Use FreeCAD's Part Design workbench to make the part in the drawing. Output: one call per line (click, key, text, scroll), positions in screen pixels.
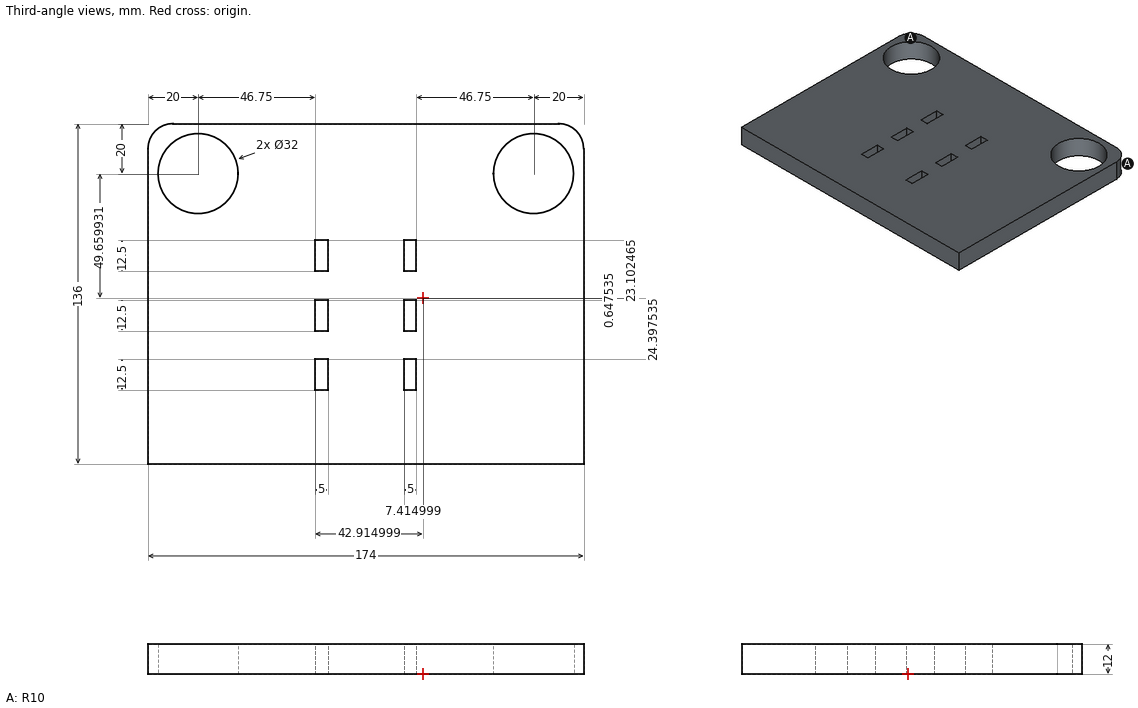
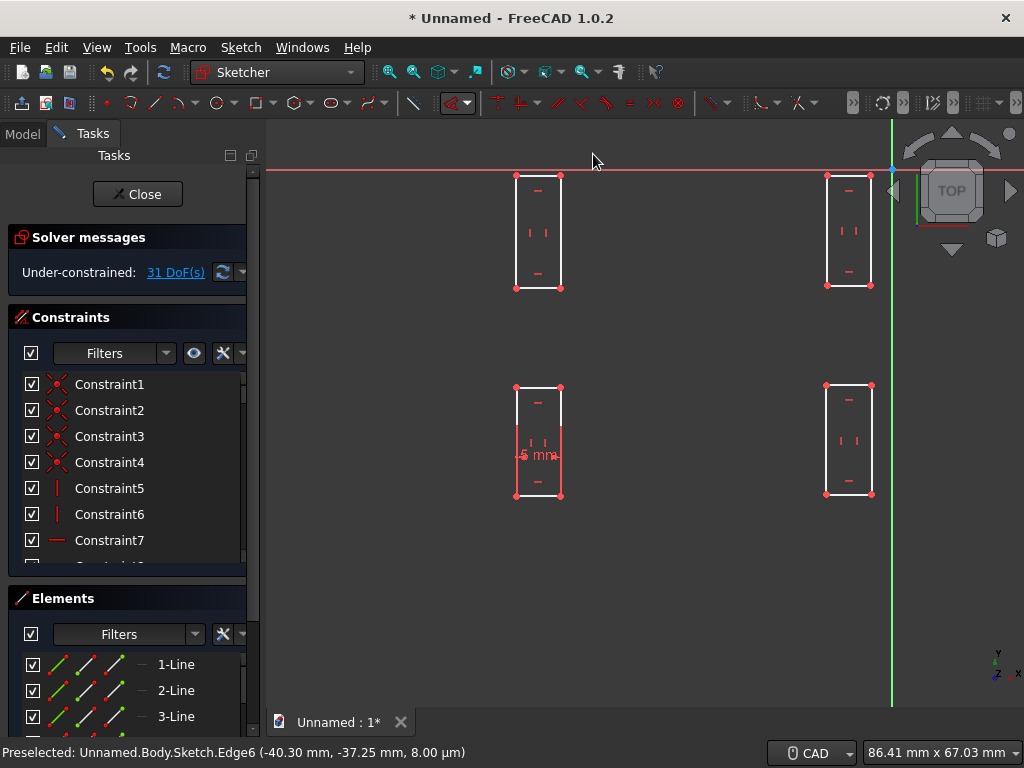
click(530, 288)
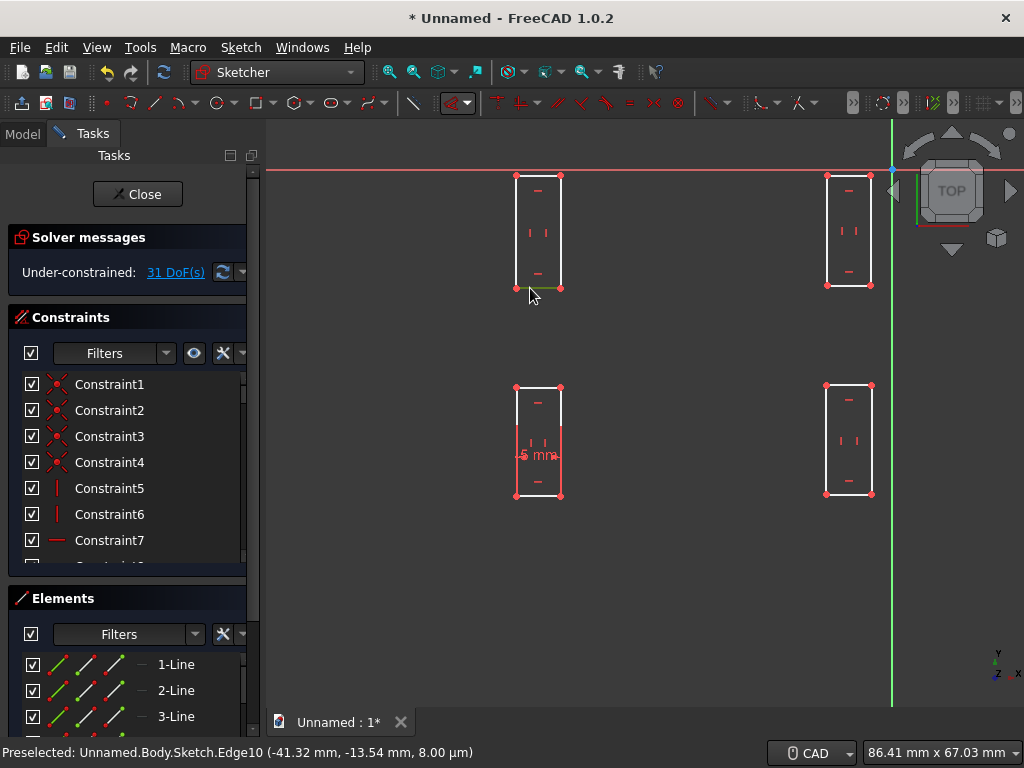
key(l)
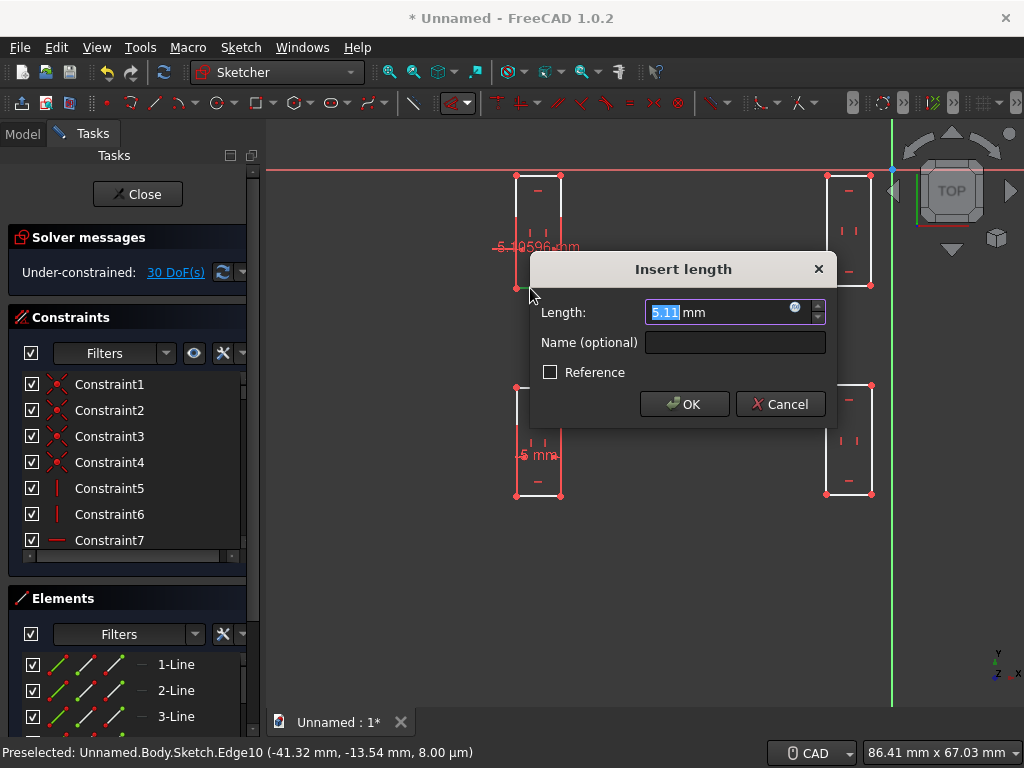
text(5)
key(Return)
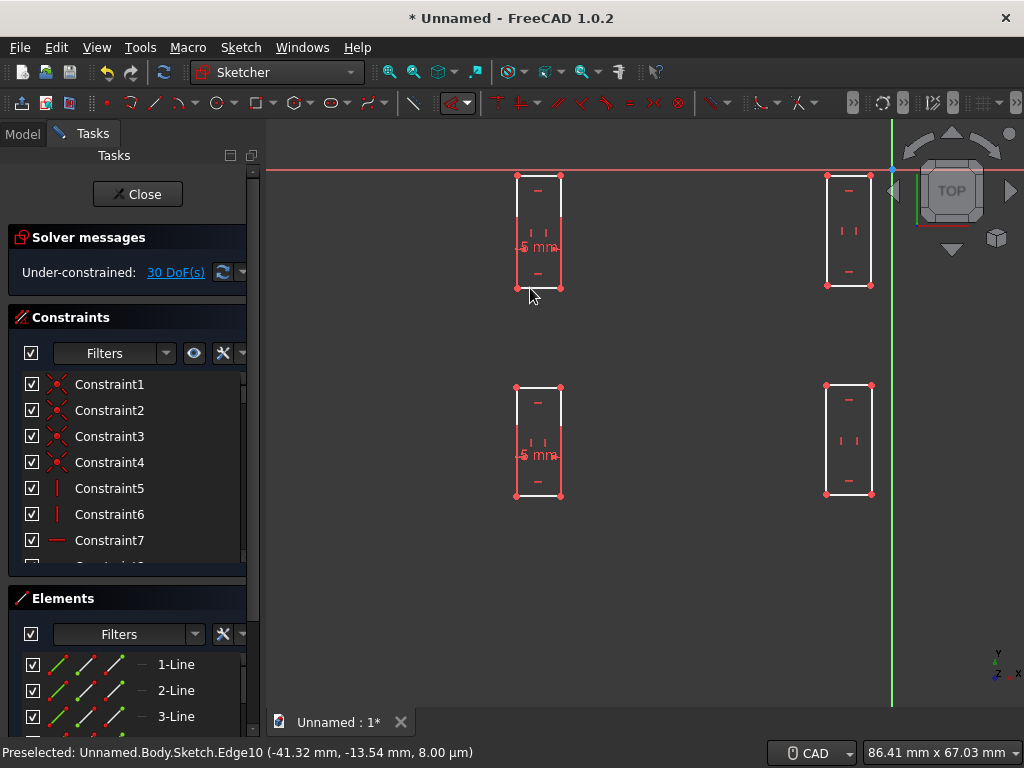
click(840, 495)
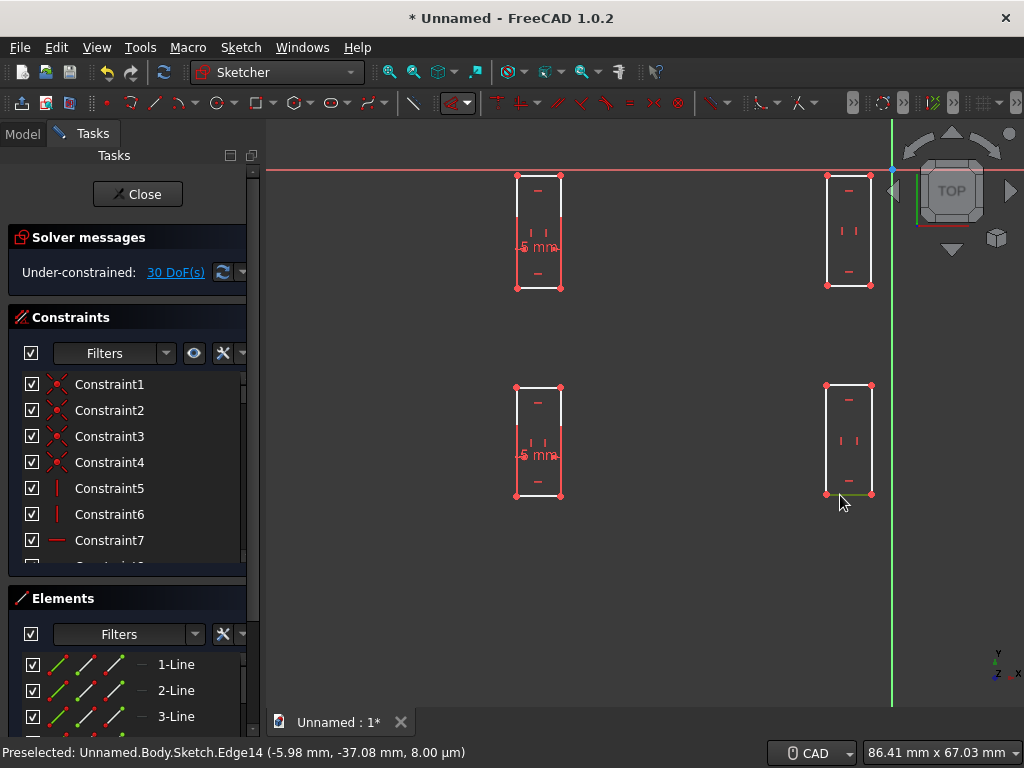
click(470, 104)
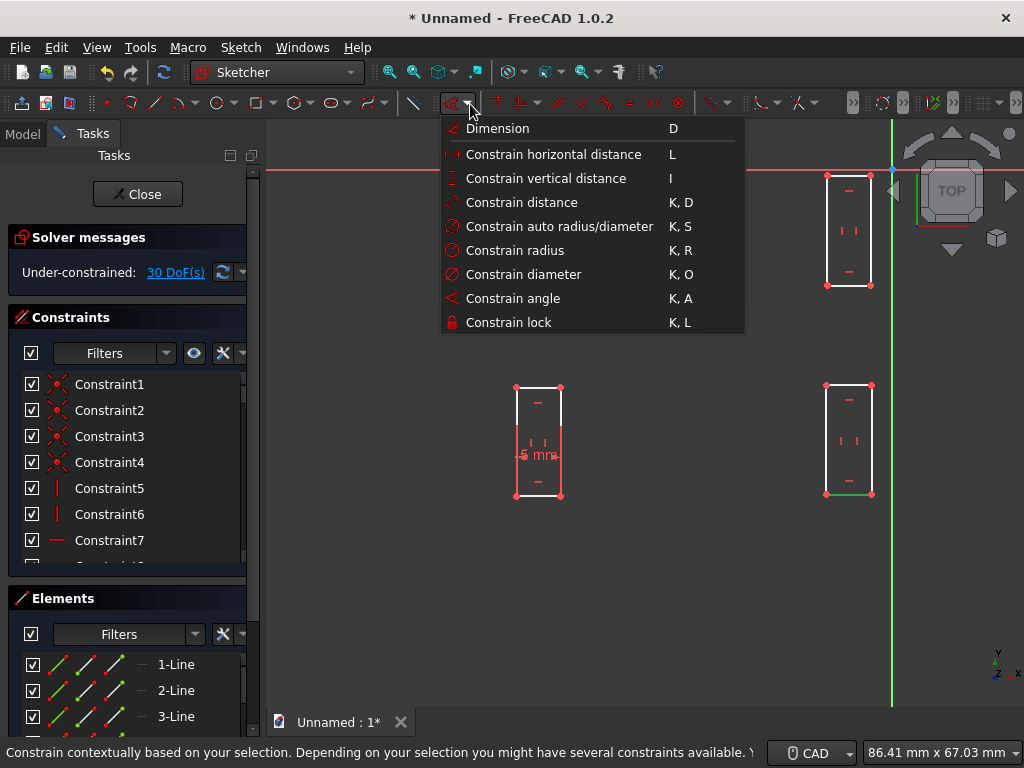
click(593, 154)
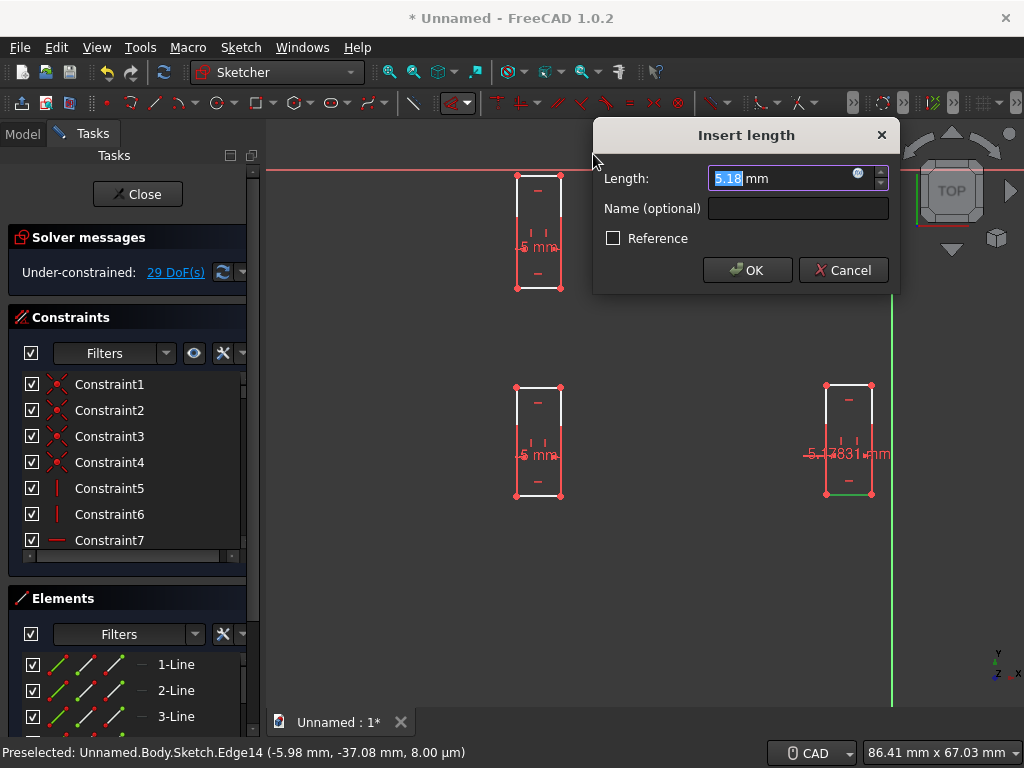
text(5)
key(Return)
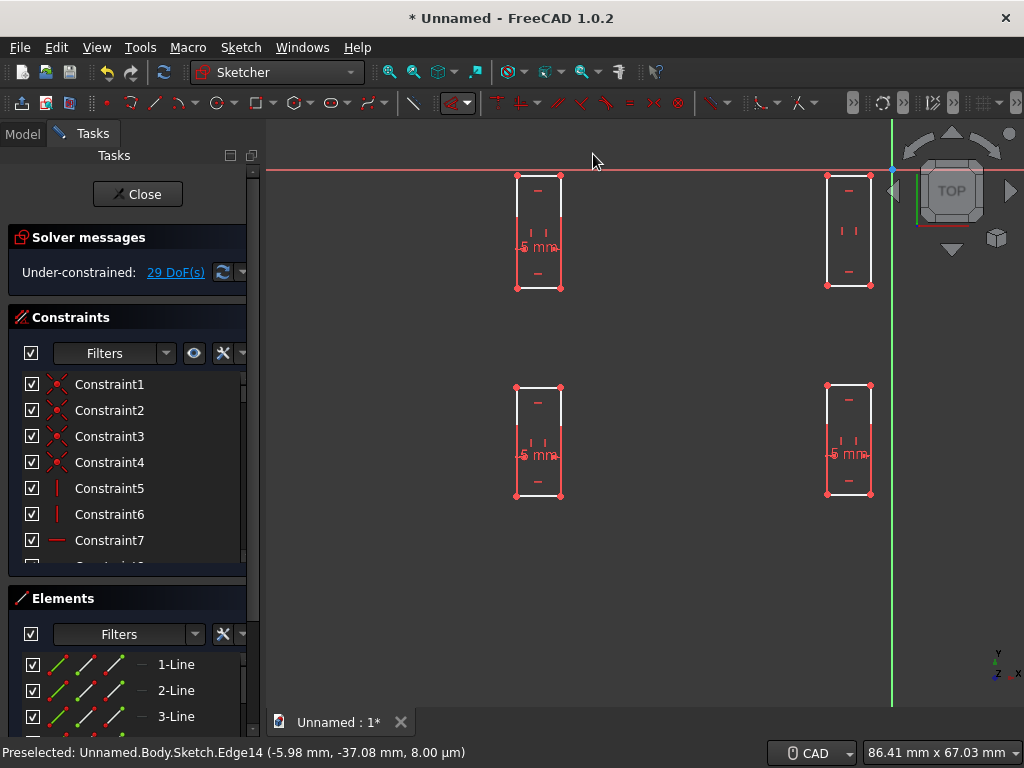
click(840, 286)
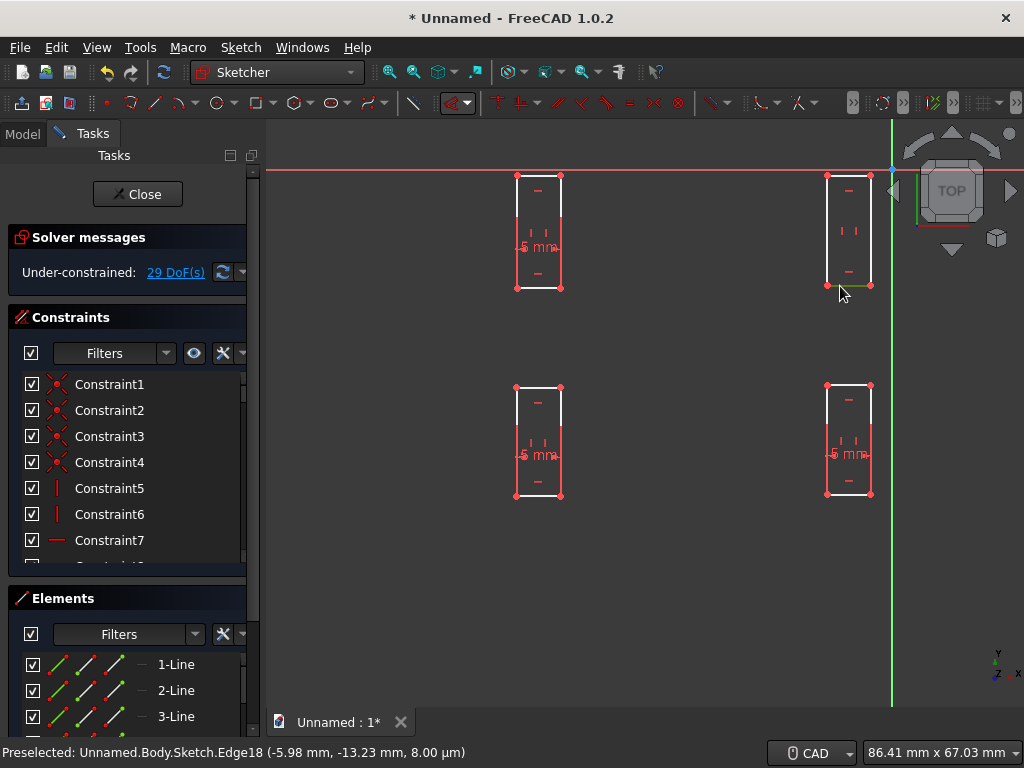
key(l)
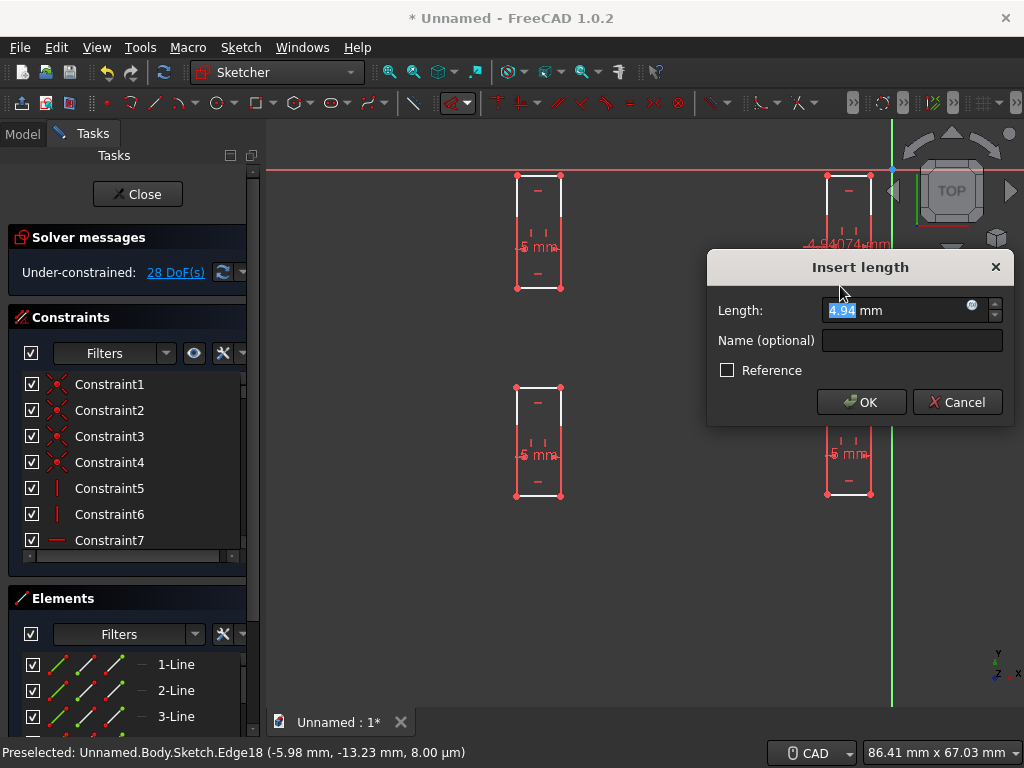
text(5)
key(Return)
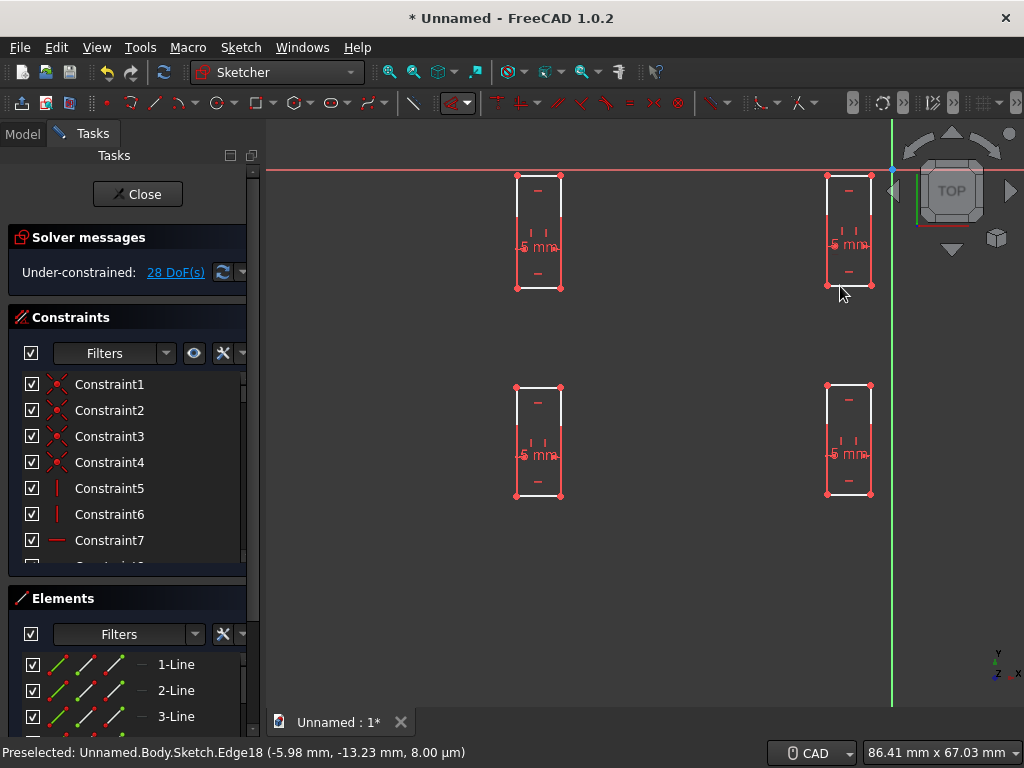
scroll(538, 497, down, 7)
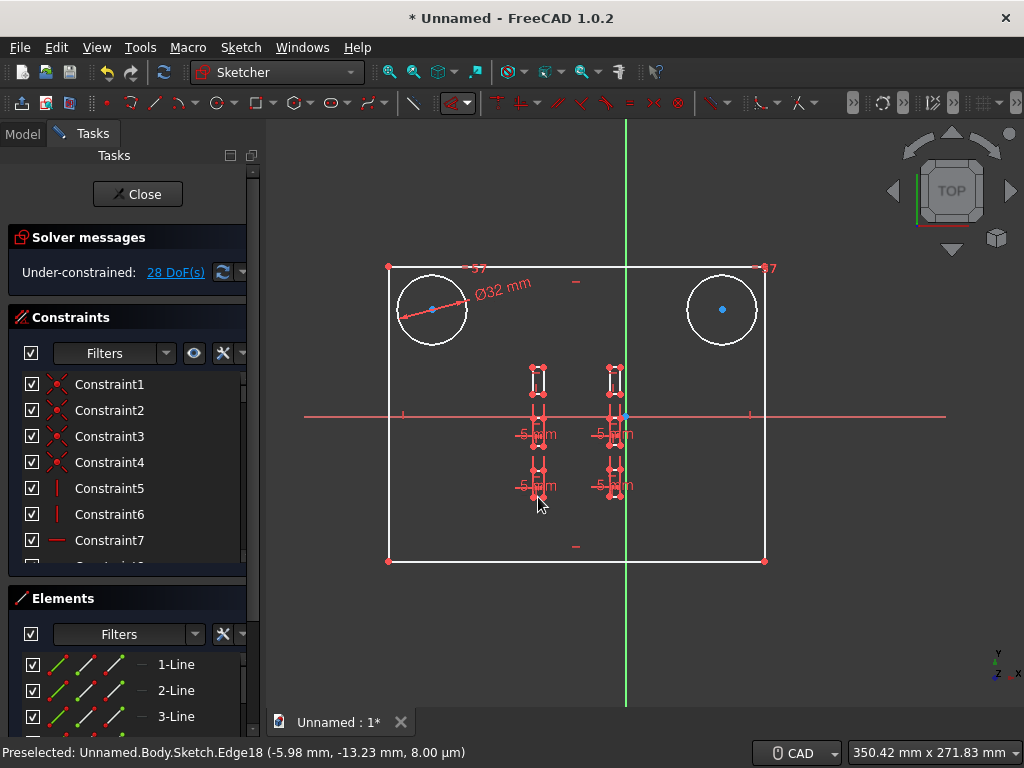
scroll(536, 394, up, 8)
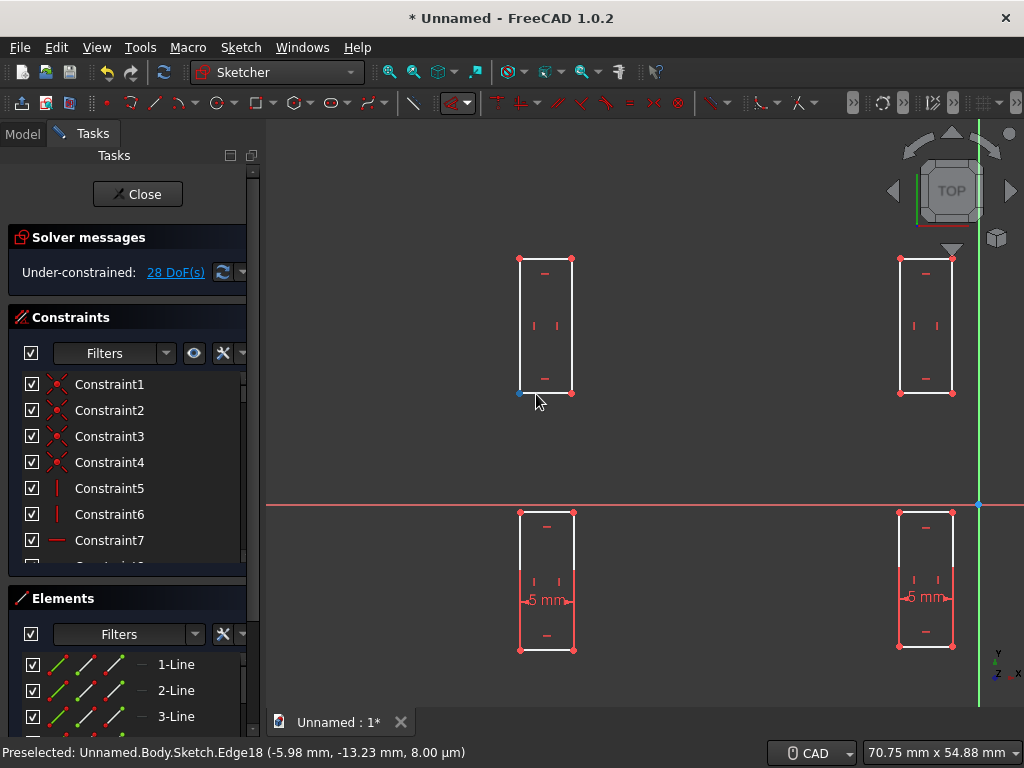
click(535, 393)